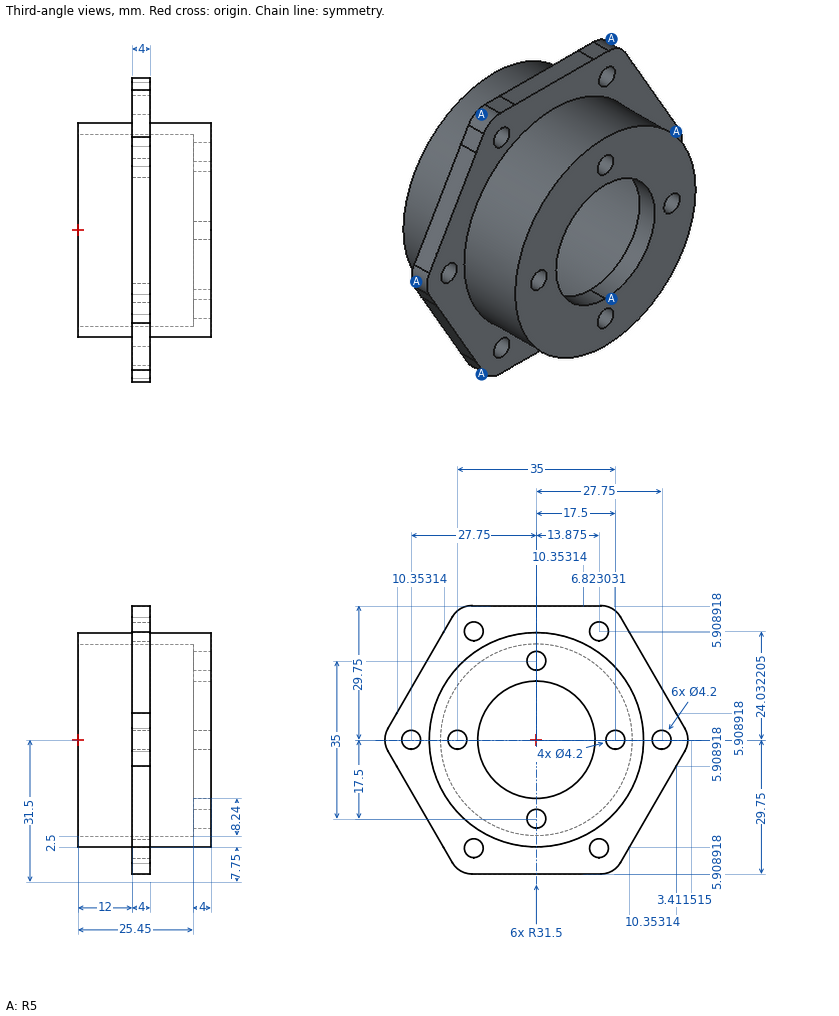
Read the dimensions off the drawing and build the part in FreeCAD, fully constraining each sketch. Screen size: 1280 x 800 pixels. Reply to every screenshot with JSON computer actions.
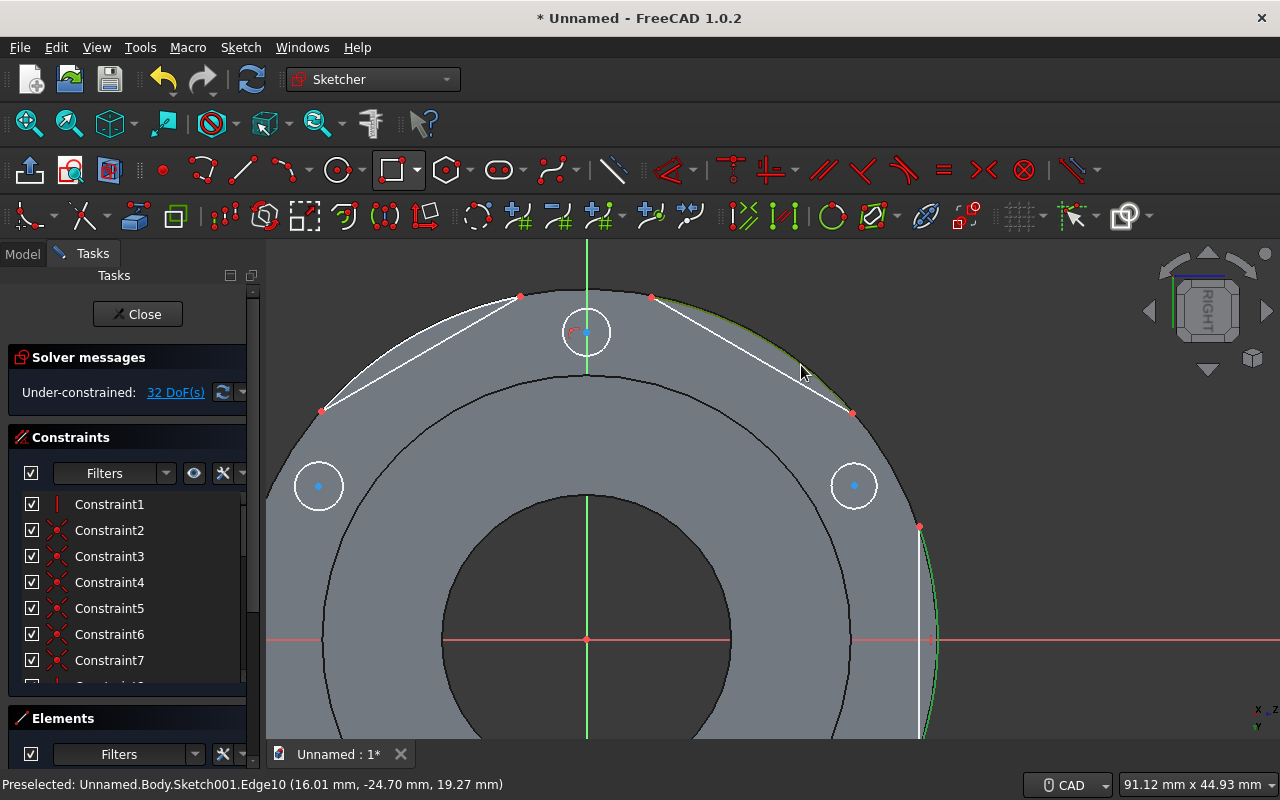
{"action": "left_click", "coordinate": [454, 317]}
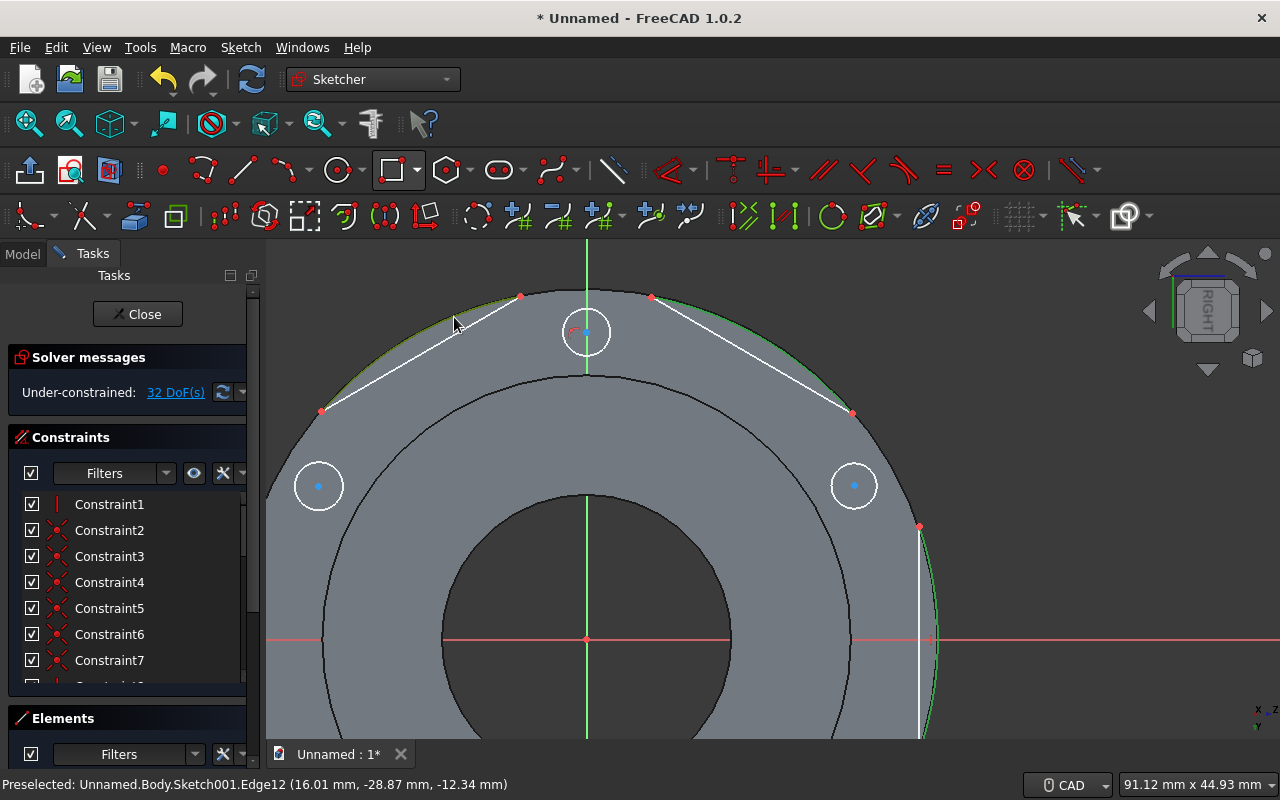
{"action": "left_click", "coordinate": [944, 170]}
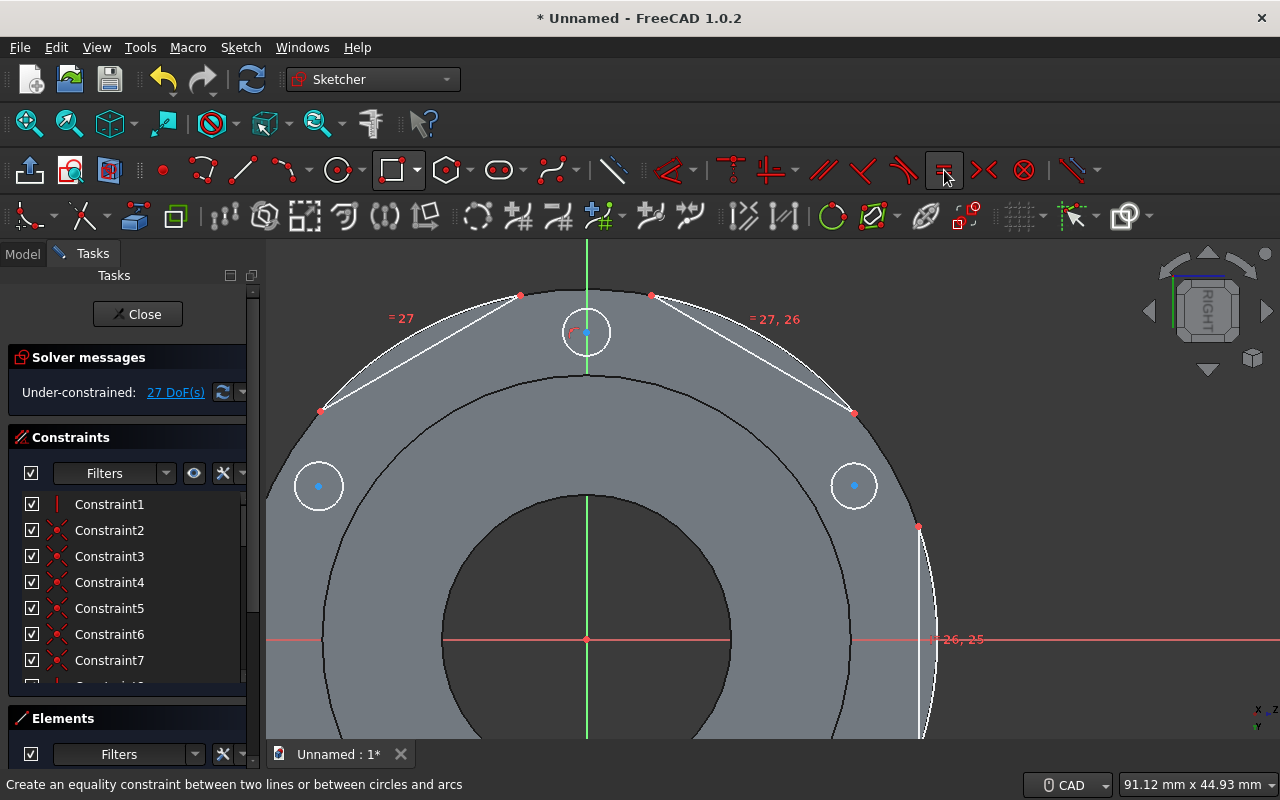
{"action": "scroll", "coordinate": [801, 366], "scroll_direction": "down", "scroll_amount": 4}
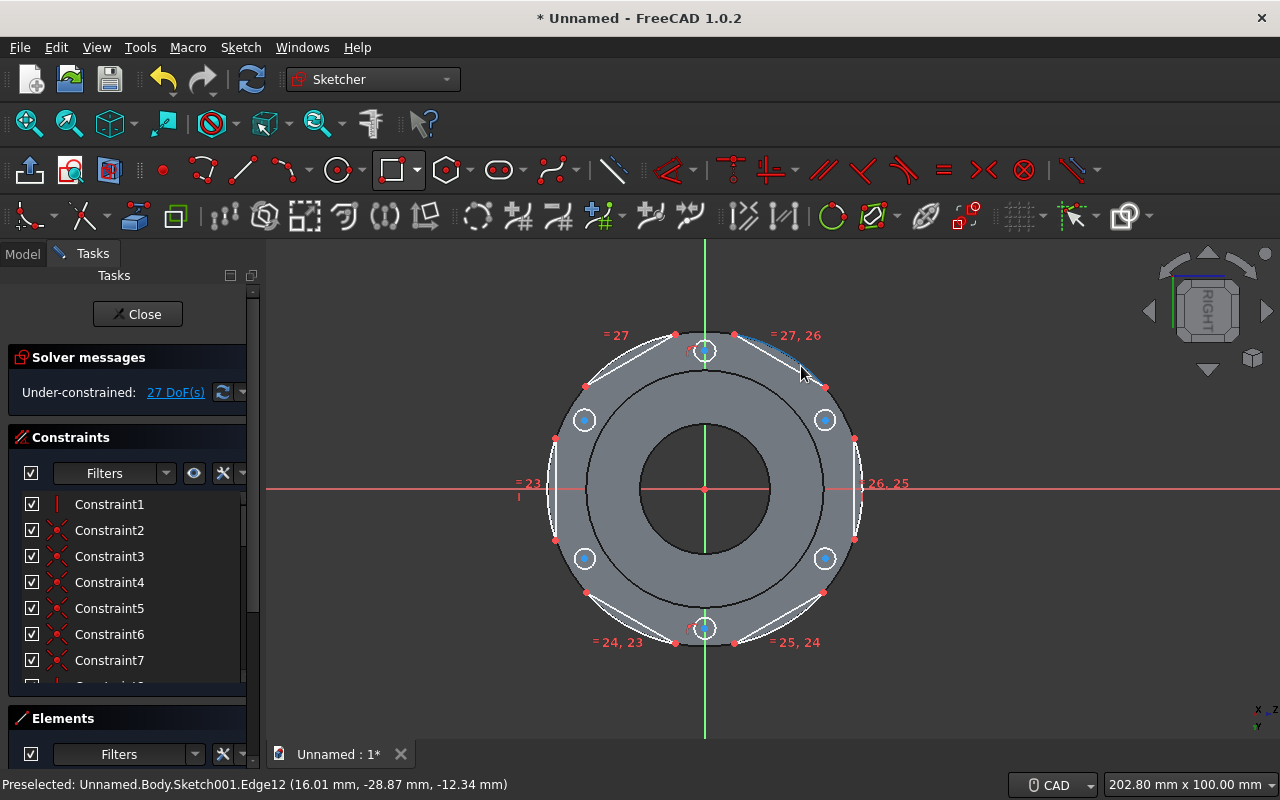
{"action": "scroll", "coordinate": [712, 621], "scroll_direction": "up", "scroll_amount": 4}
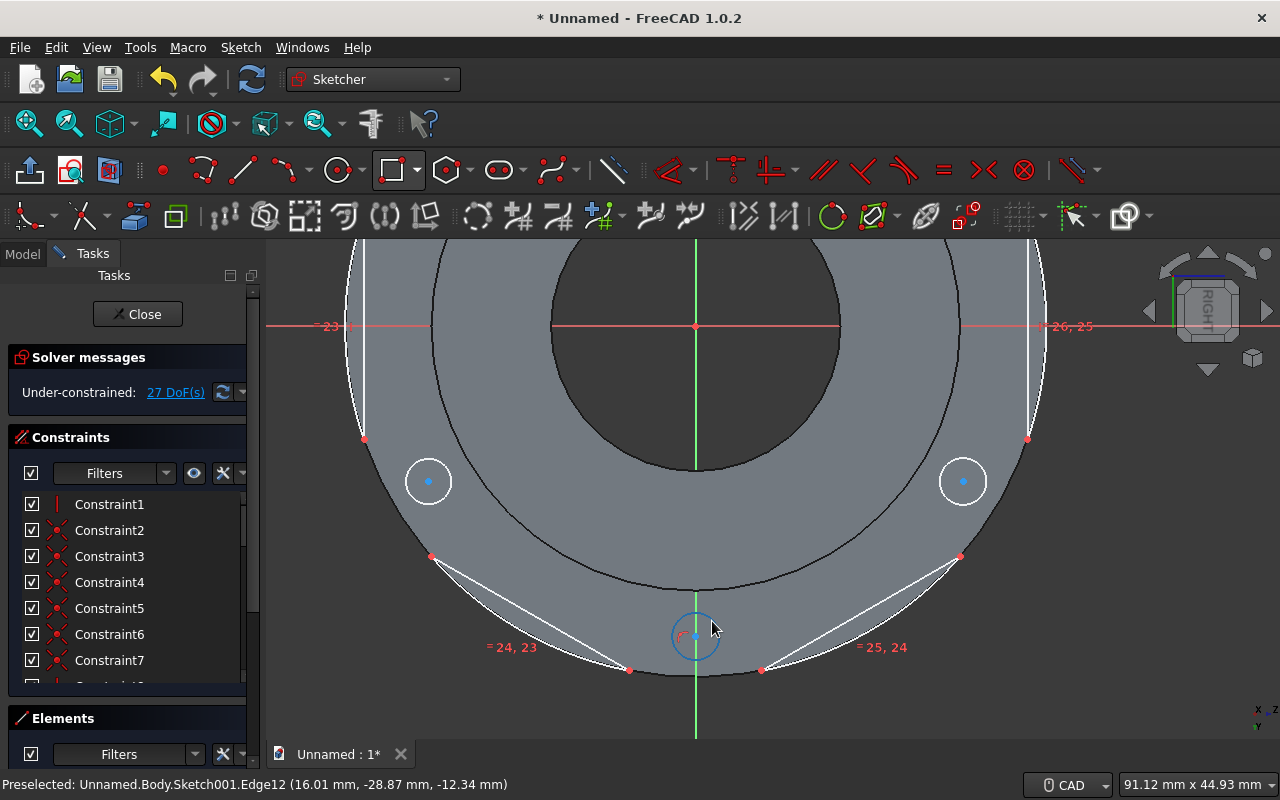
{"action": "left_click", "coordinate": [712, 620]}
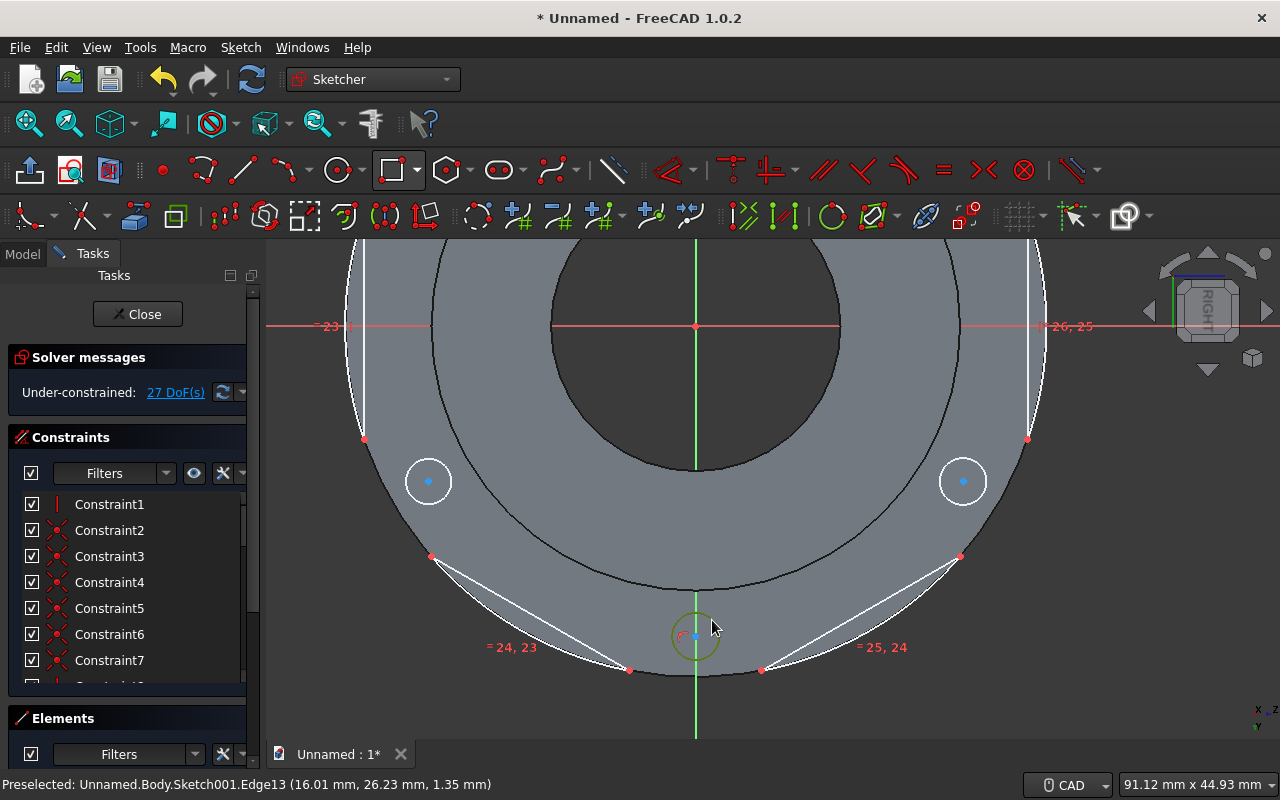
{"action": "left_click", "coordinate": [980, 465]}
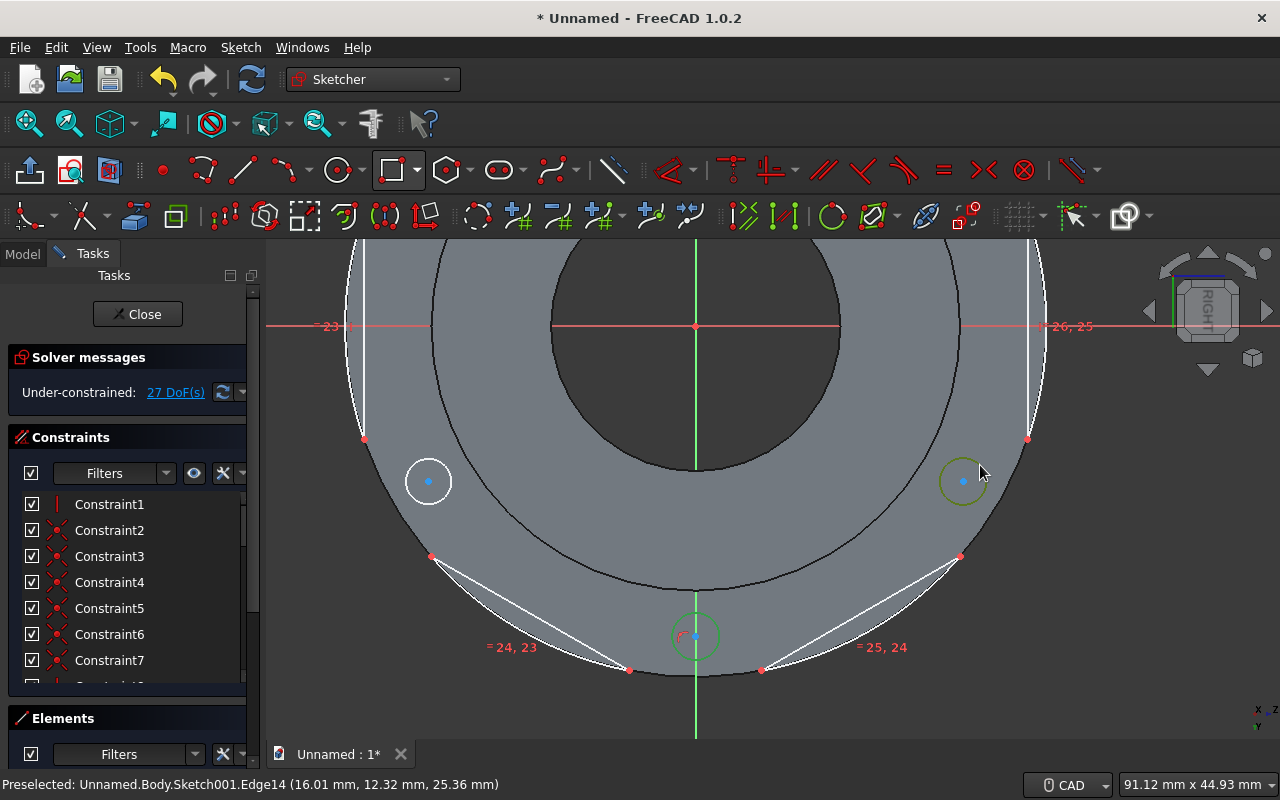
{"action": "scroll", "coordinate": [712, 622], "scroll_direction": "down", "scroll_amount": 4}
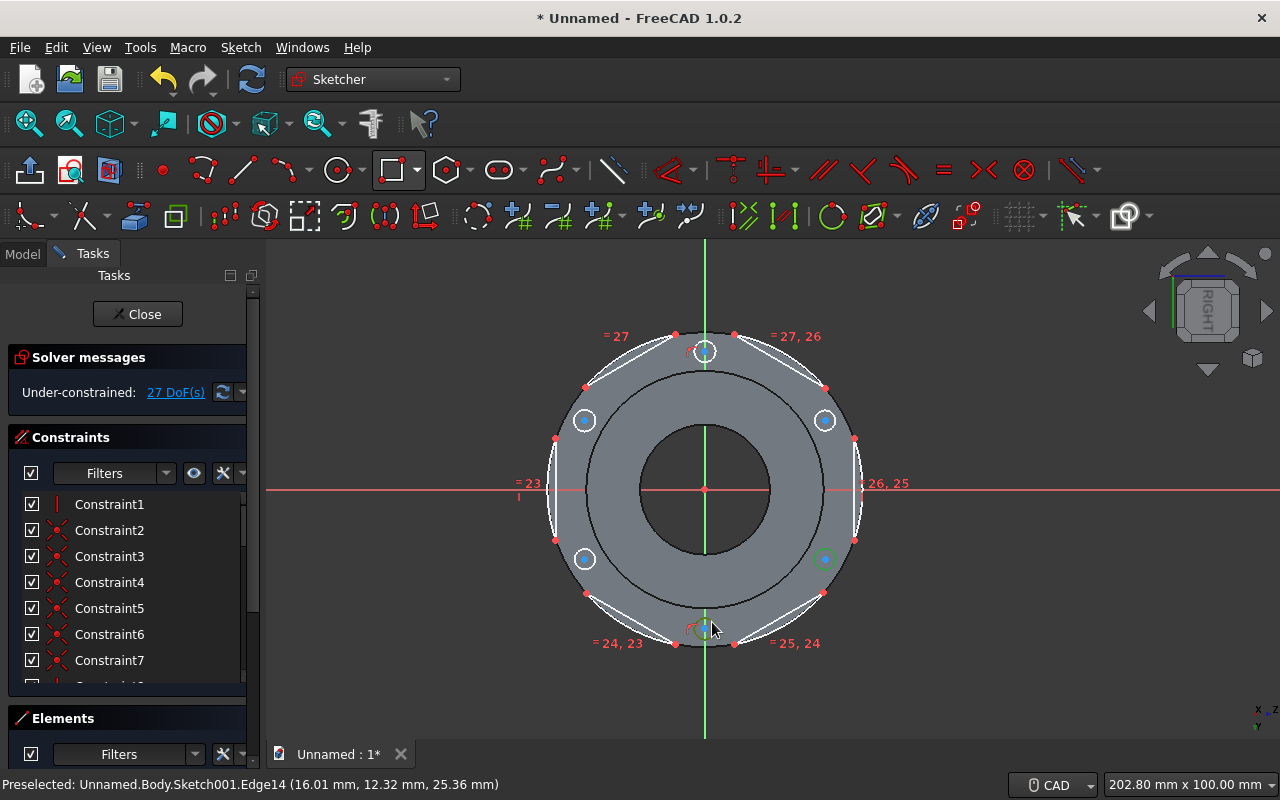
{"action": "scroll", "coordinate": [832, 413], "scroll_direction": "up", "scroll_amount": 2}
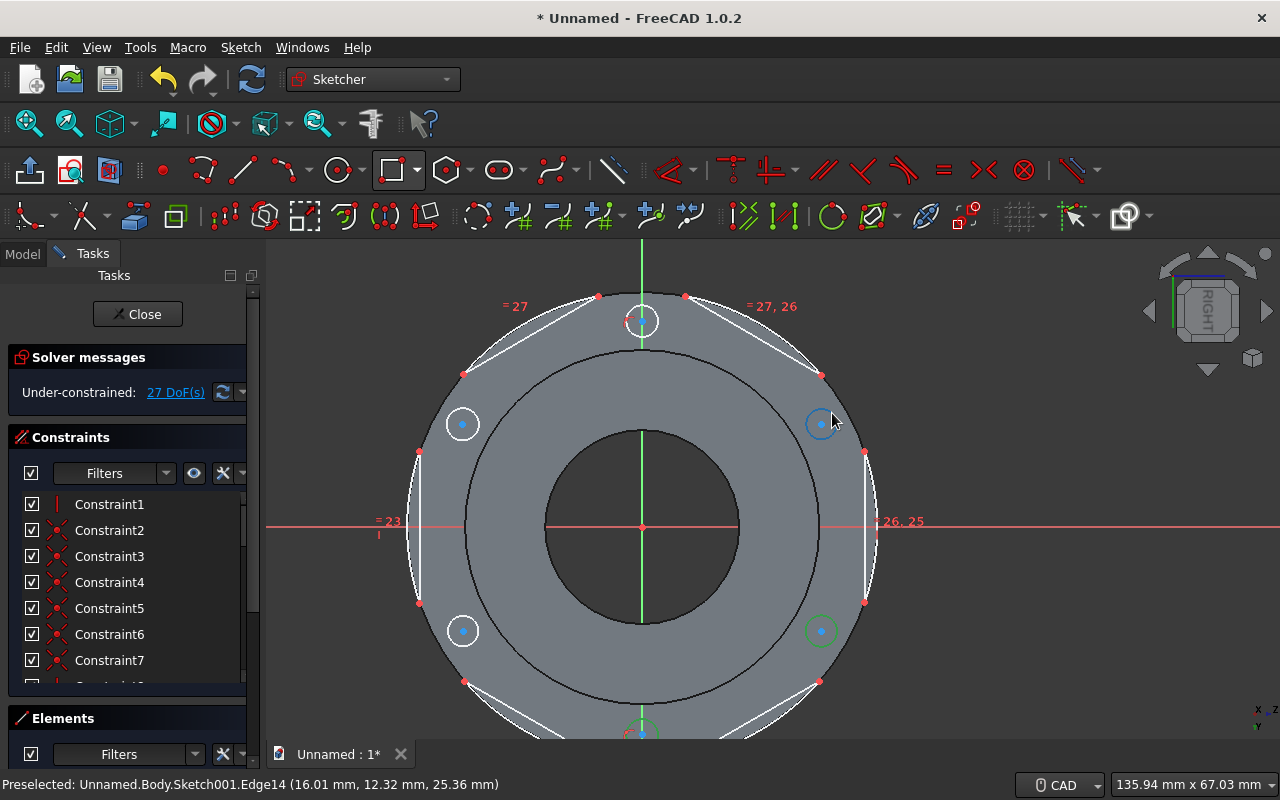
{"action": "left_click", "coordinate": [832, 413]}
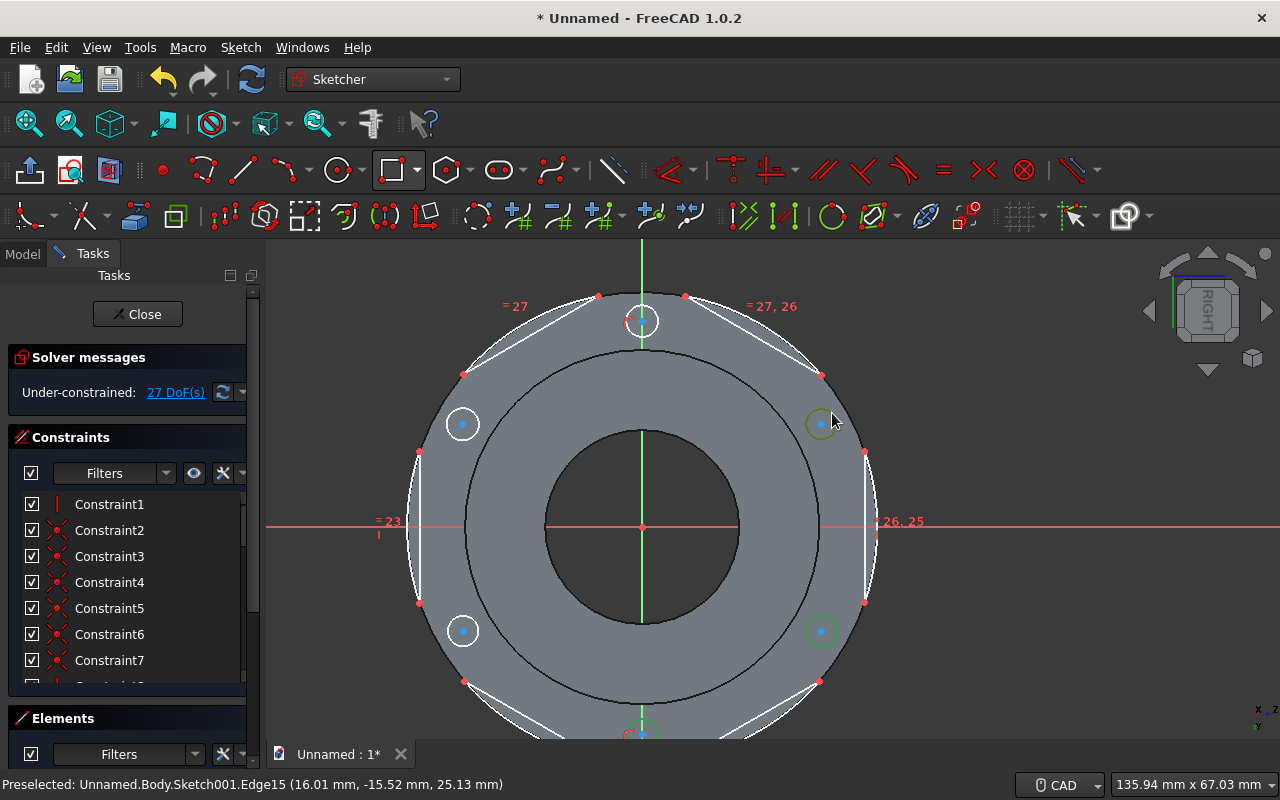
{"action": "scroll", "coordinate": [653, 310], "scroll_direction": "up", "scroll_amount": 2}